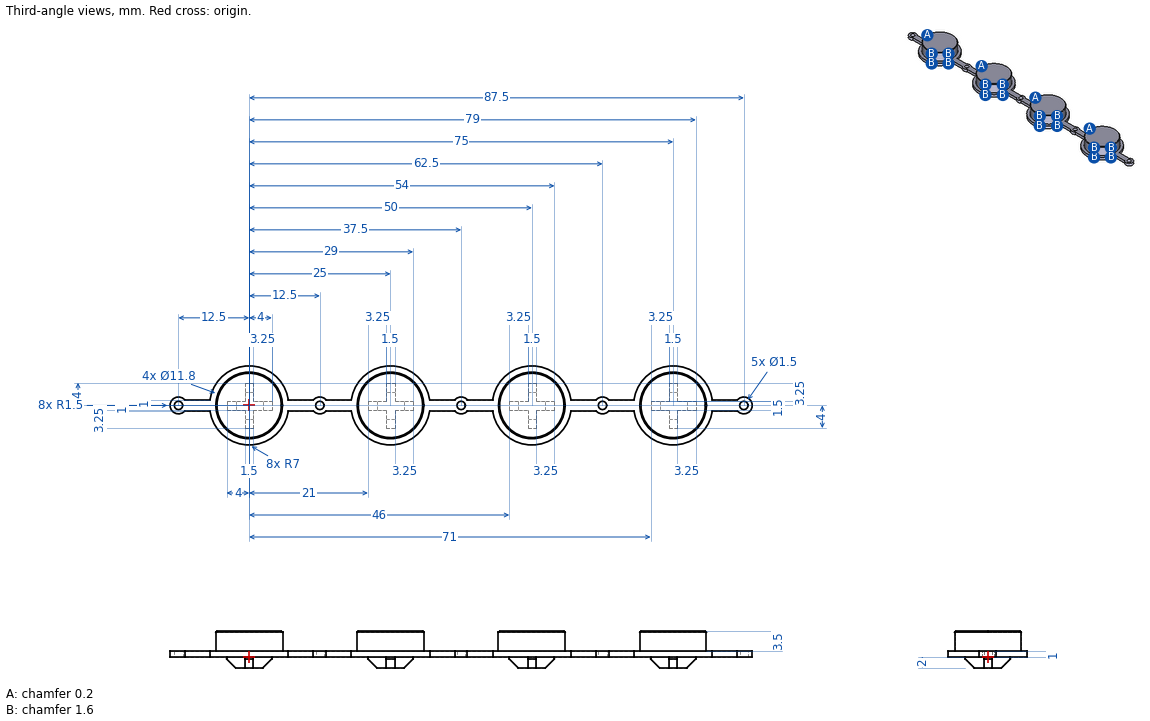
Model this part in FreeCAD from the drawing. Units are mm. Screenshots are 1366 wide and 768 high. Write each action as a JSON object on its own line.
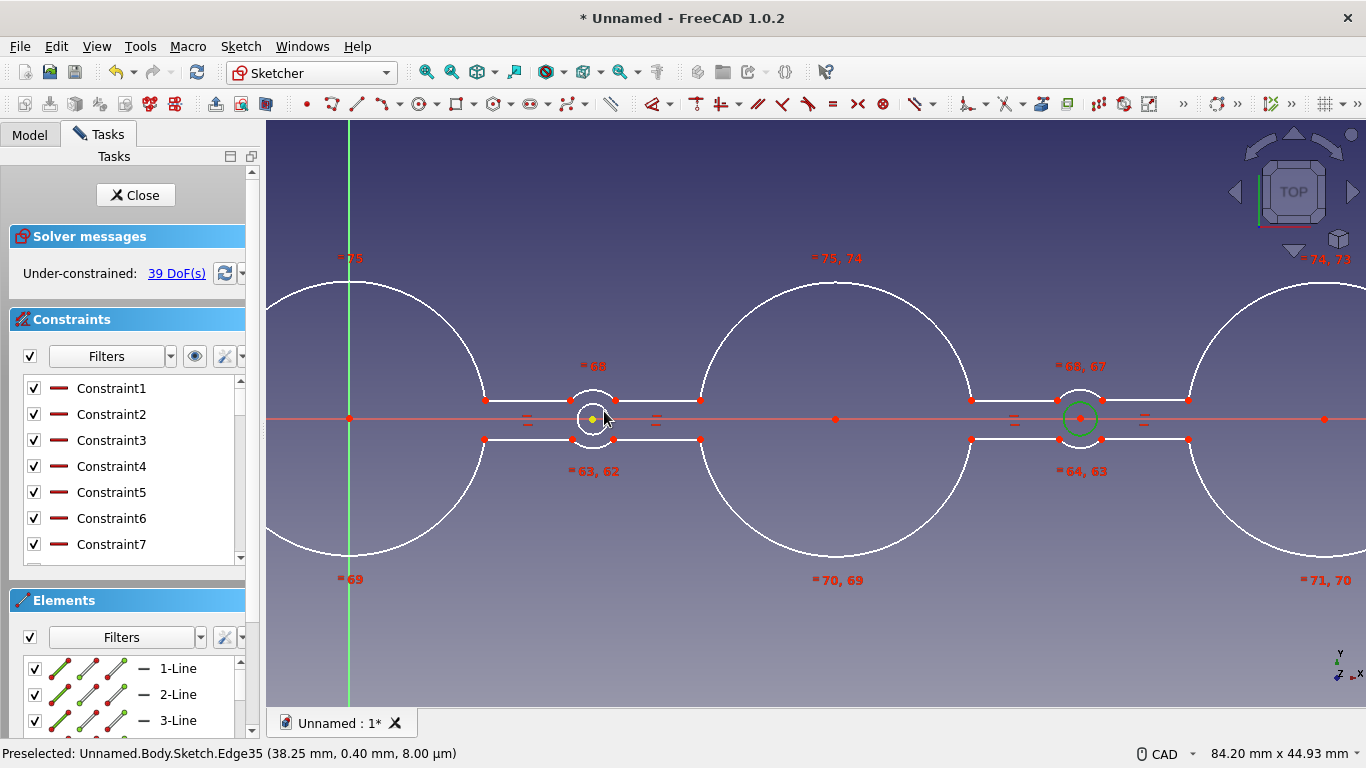
{"action": "left_click", "coordinate": [604, 407]}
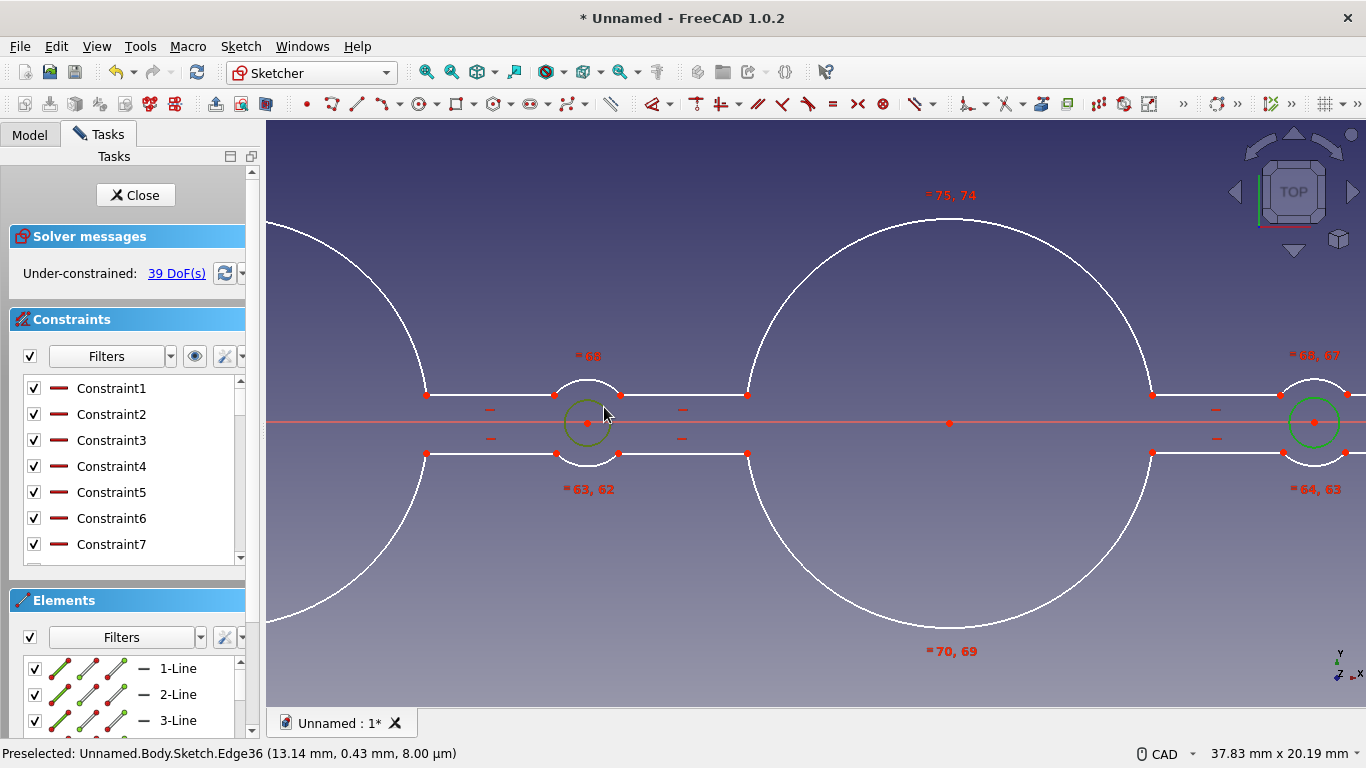
{"action": "scroll", "coordinate": [604, 411], "scroll_direction": "down", "scroll_amount": 8}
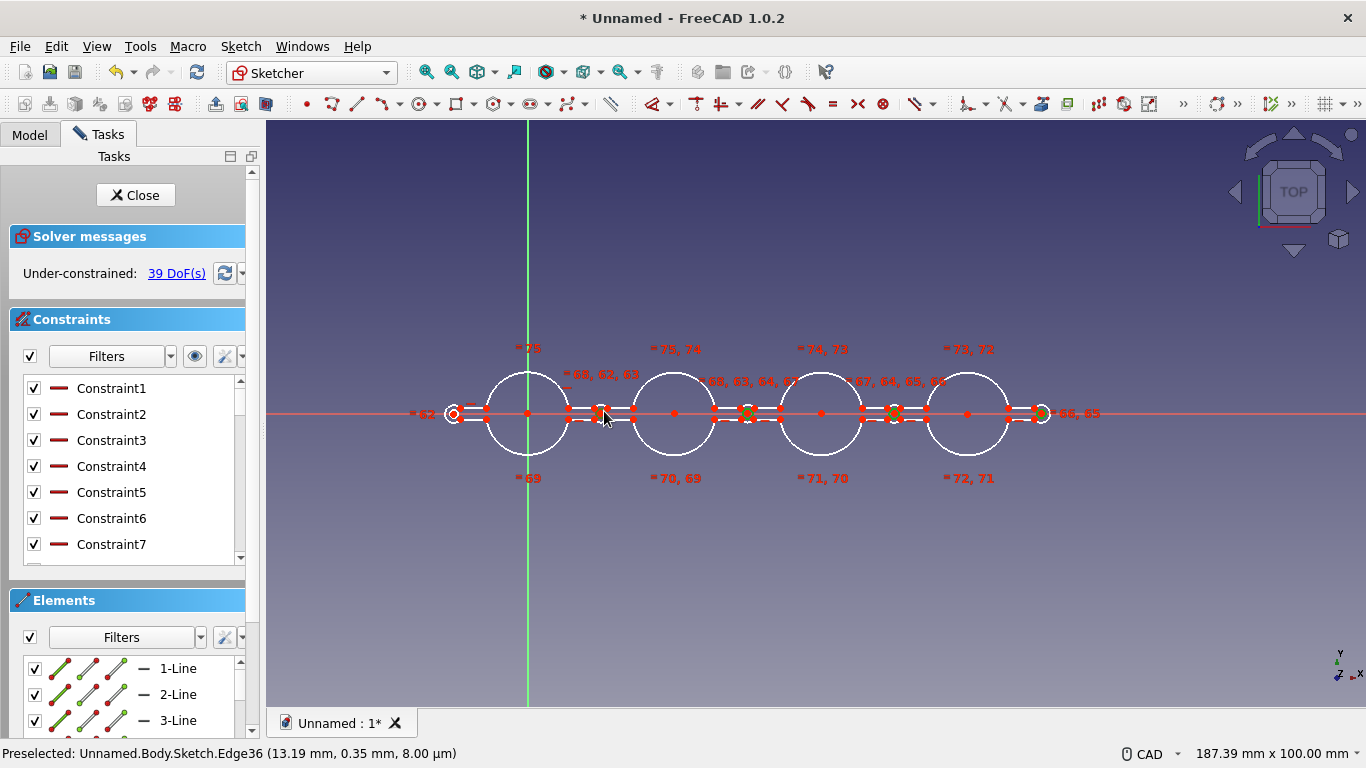
{"action": "scroll", "coordinate": [457, 411], "scroll_direction": "up", "scroll_amount": 9}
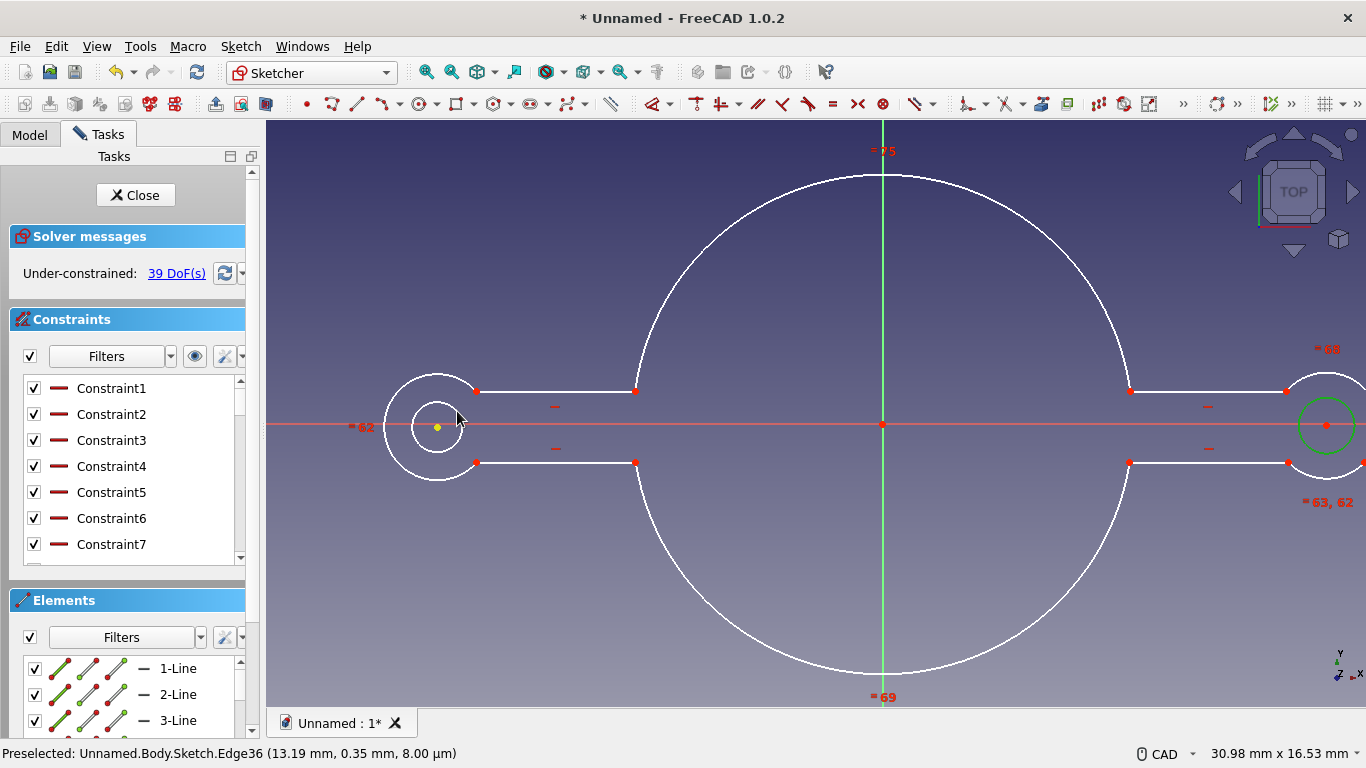
{"action": "left_click", "coordinate": [455, 409]}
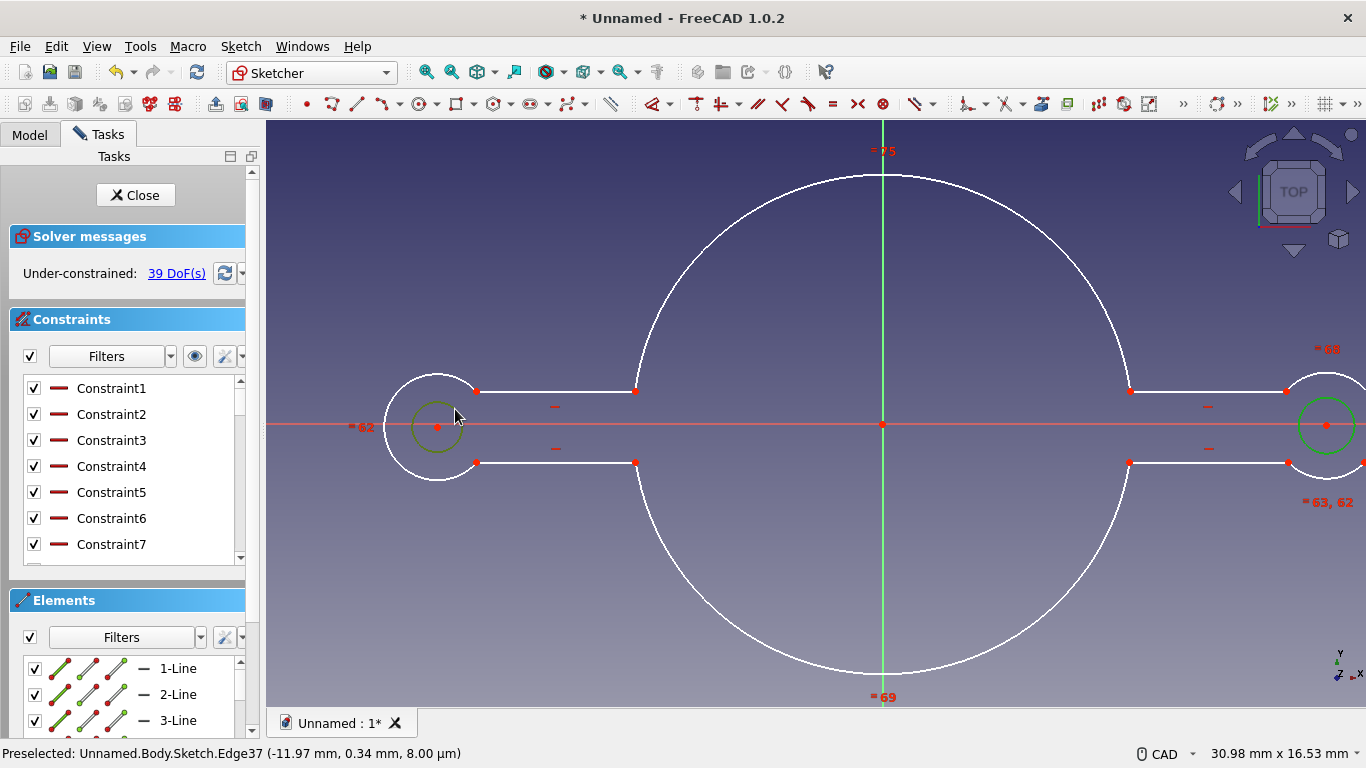
{"action": "left_click", "coordinate": [833, 104]}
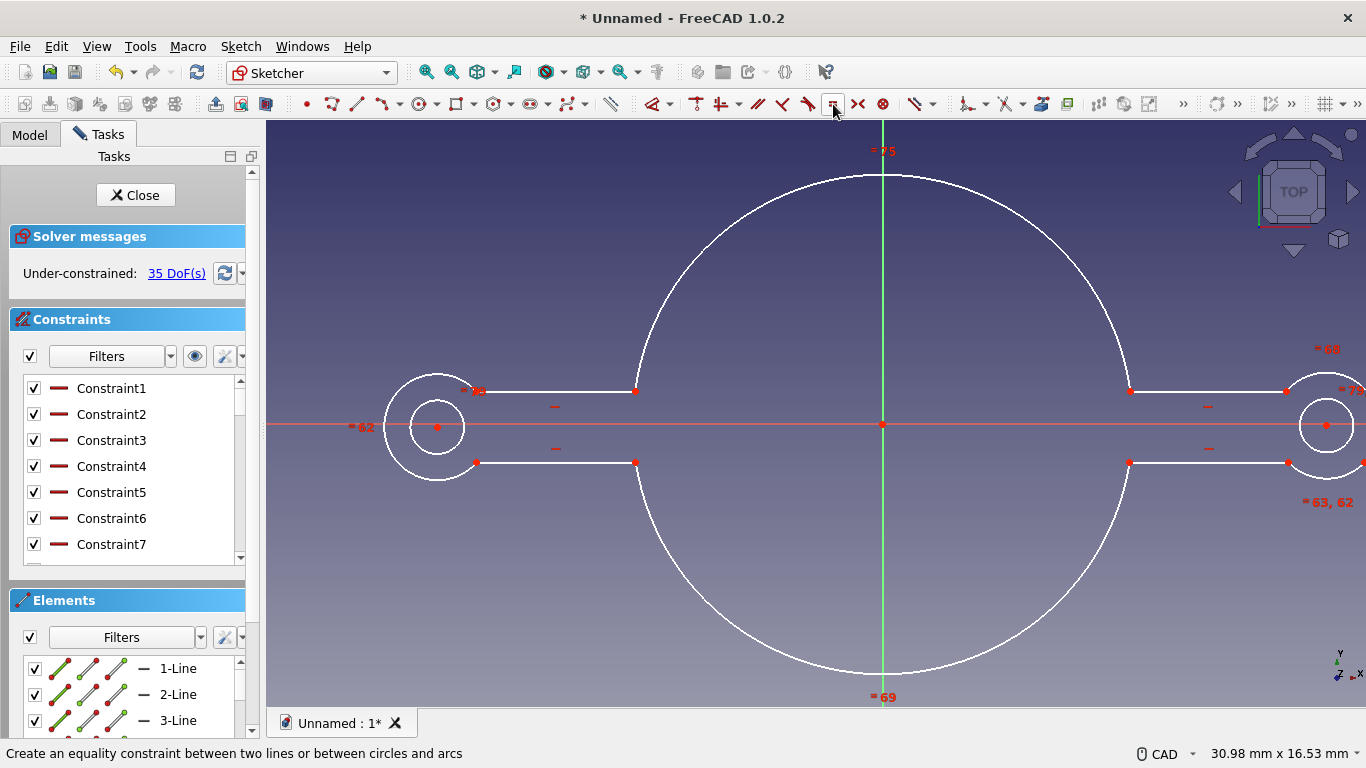
{"action": "scroll", "coordinate": [457, 411], "scroll_direction": "down", "scroll_amount": 9}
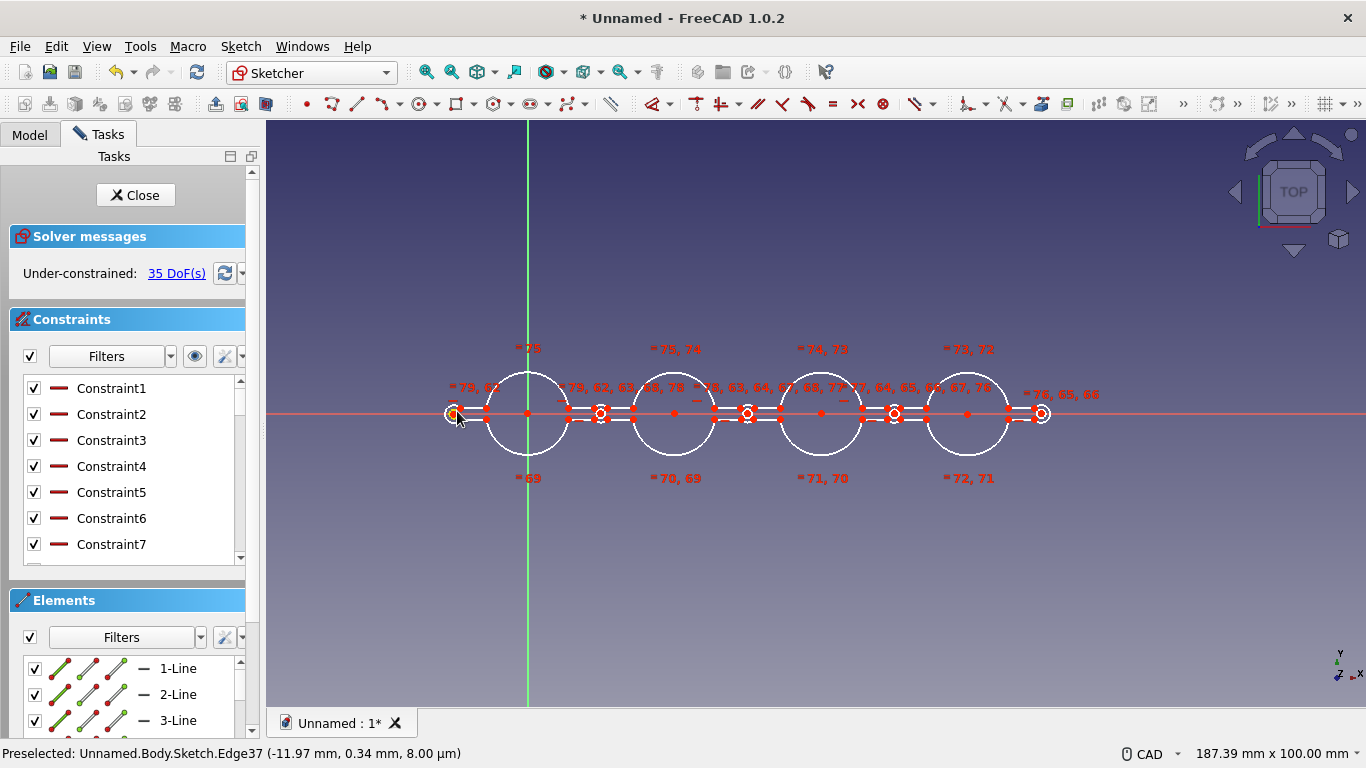
{"action": "scroll", "coordinate": [454, 414], "scroll_direction": "up", "scroll_amount": 2}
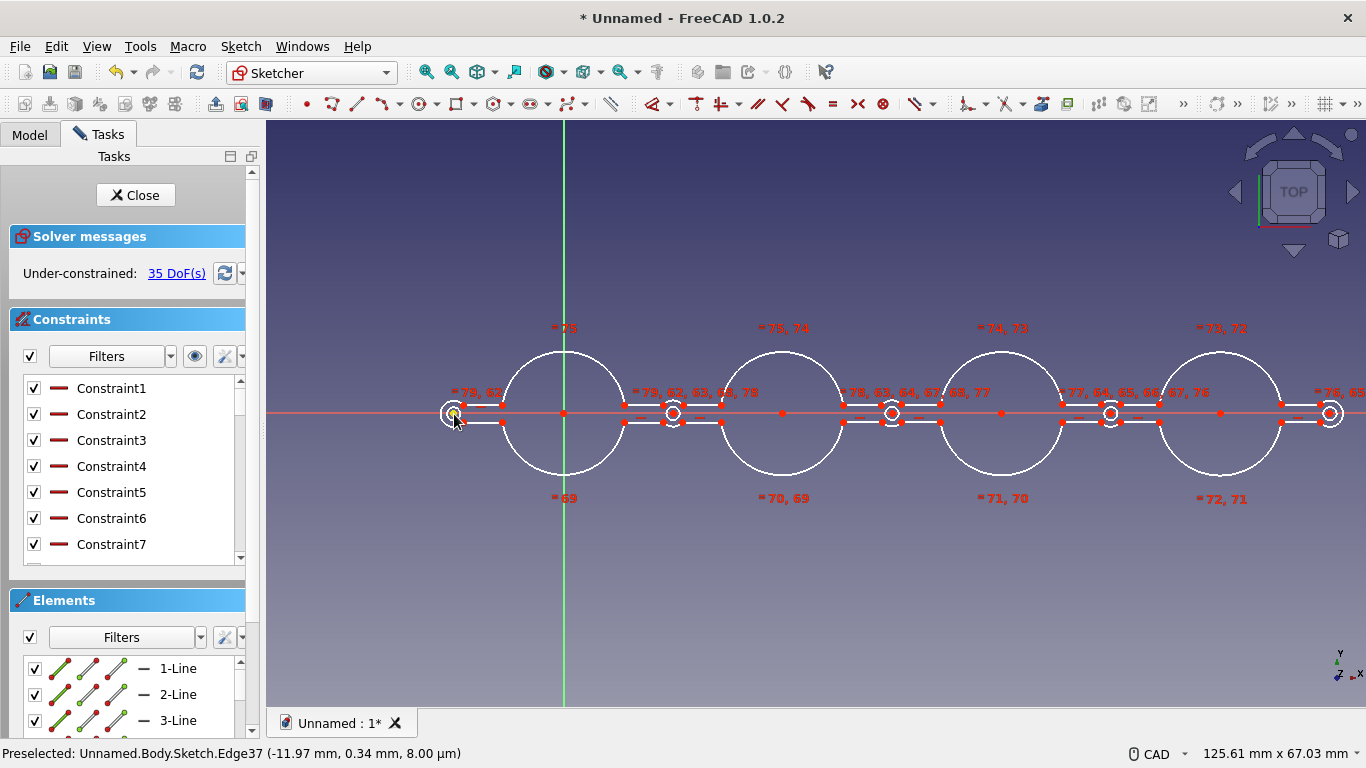
{"action": "left_click", "coordinate": [454, 414]}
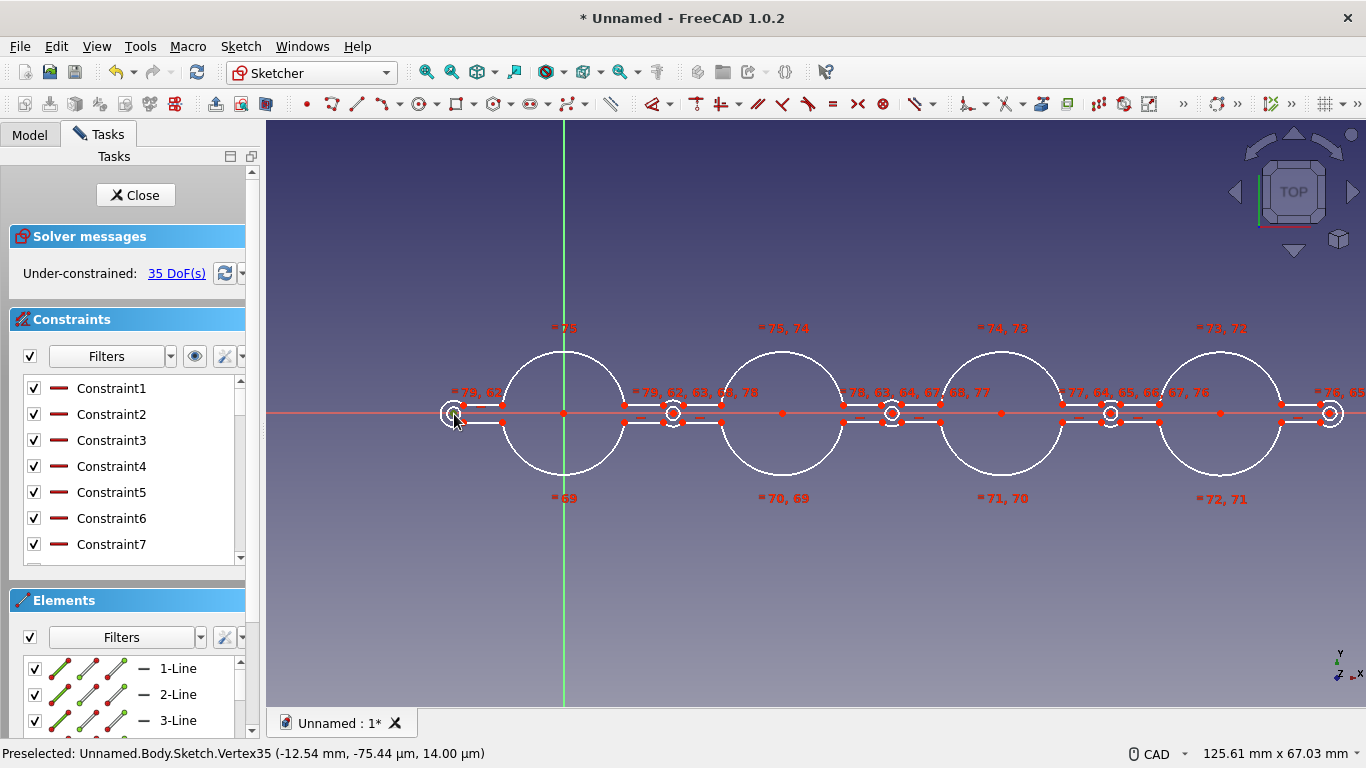
{"action": "left_click", "coordinate": [359, 413]}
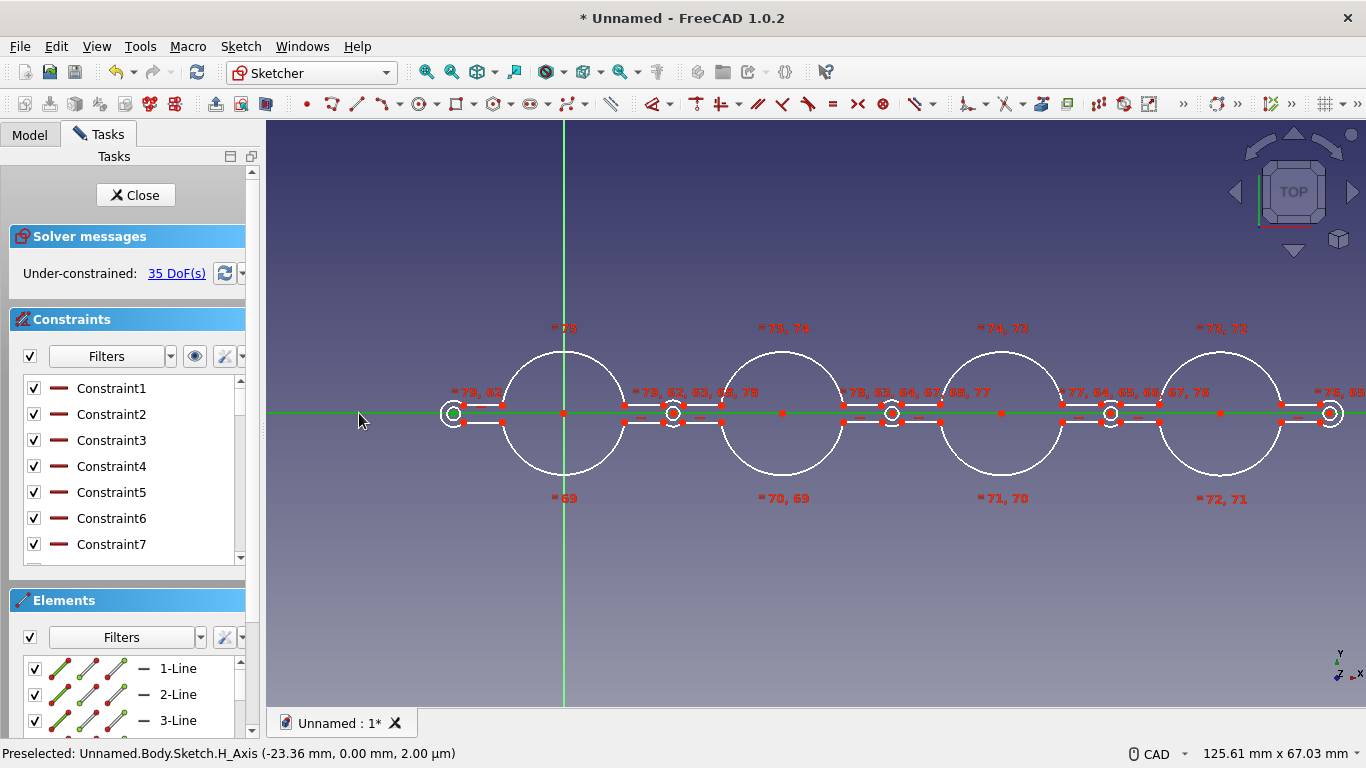
{"action": "key", "text": "c"}